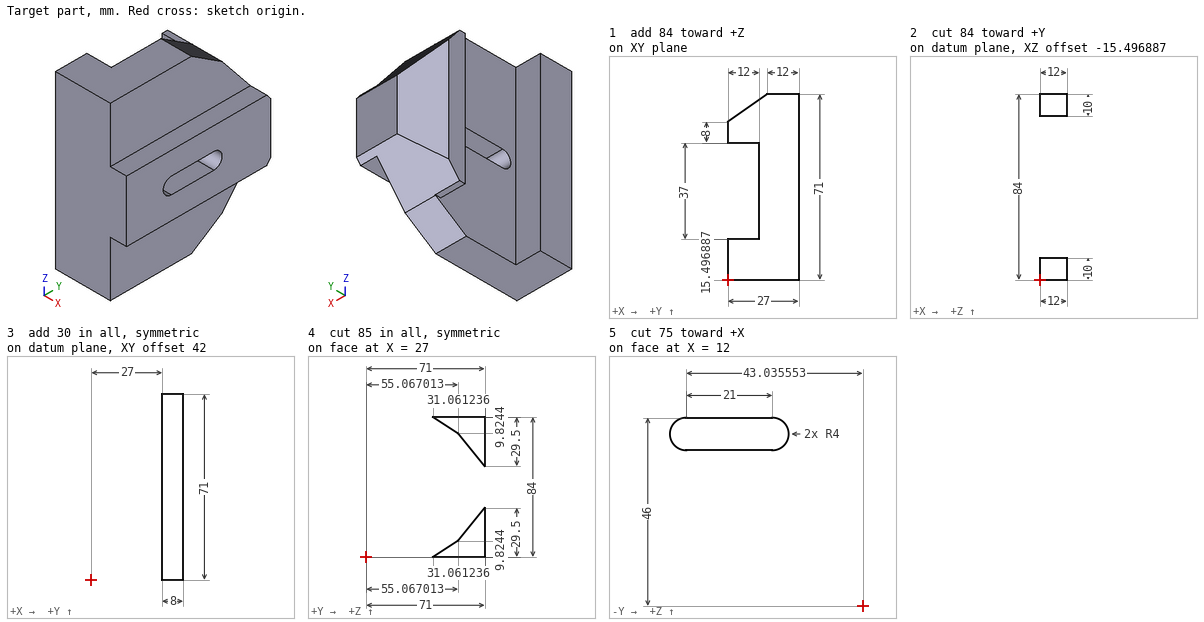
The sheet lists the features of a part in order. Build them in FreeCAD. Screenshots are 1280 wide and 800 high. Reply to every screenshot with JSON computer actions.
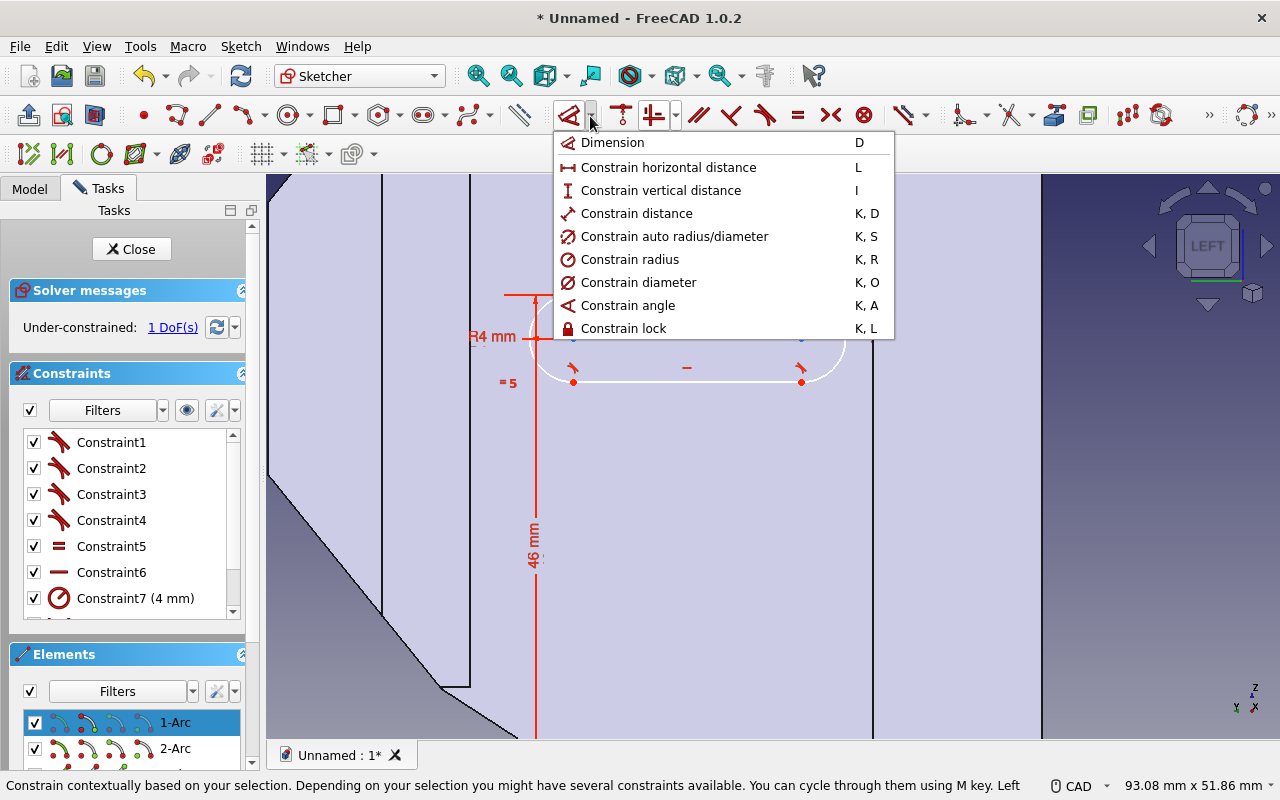
{"action": "left_click", "coordinate": [724, 168]}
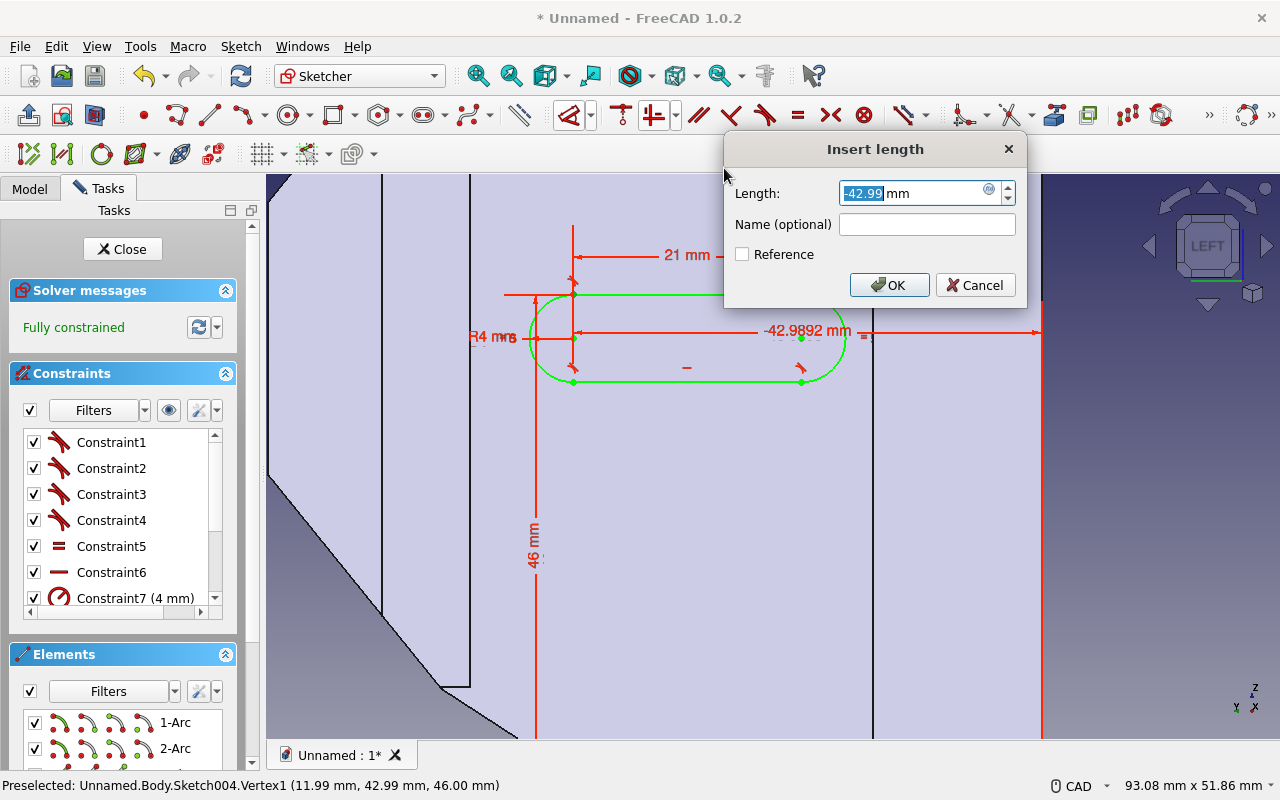
{"action": "type", "text": "-43.035553"}
{"action": "key", "text": "Return"}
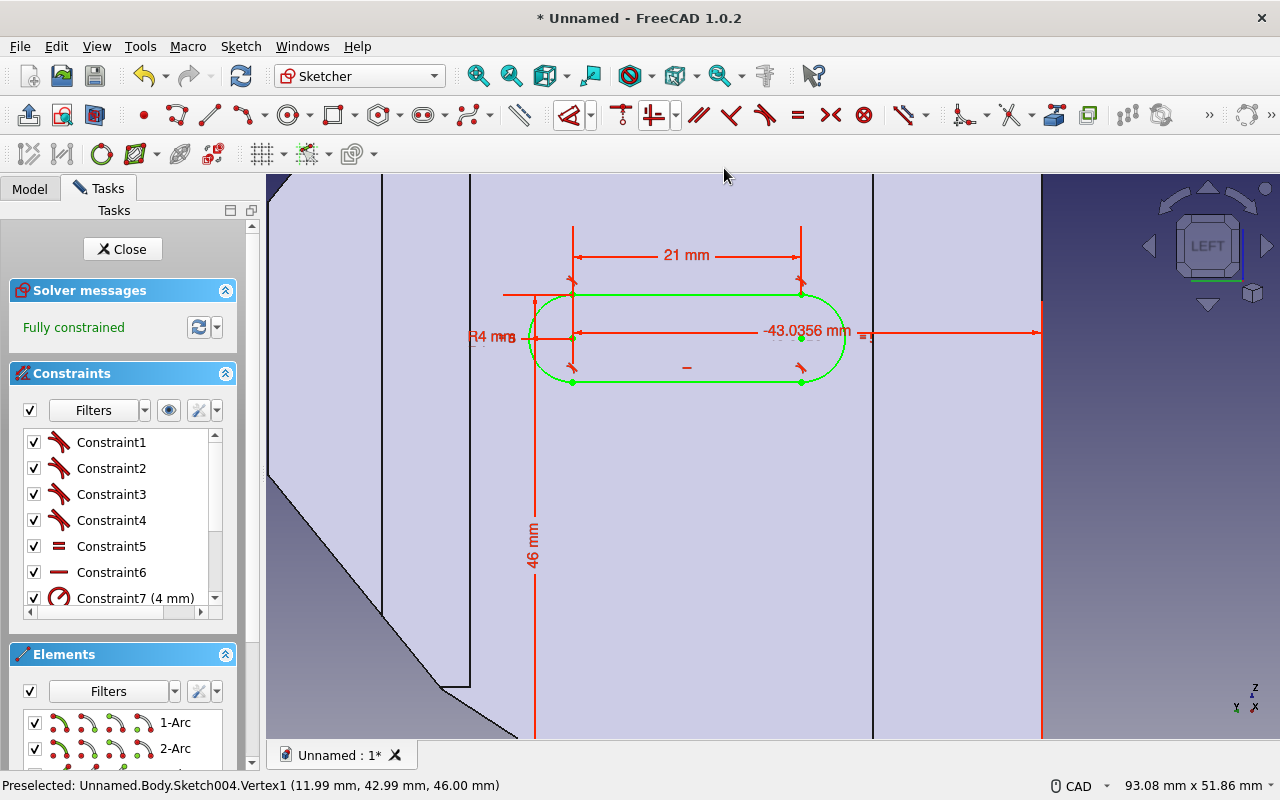
{"action": "left_click", "coordinate": [123, 249]}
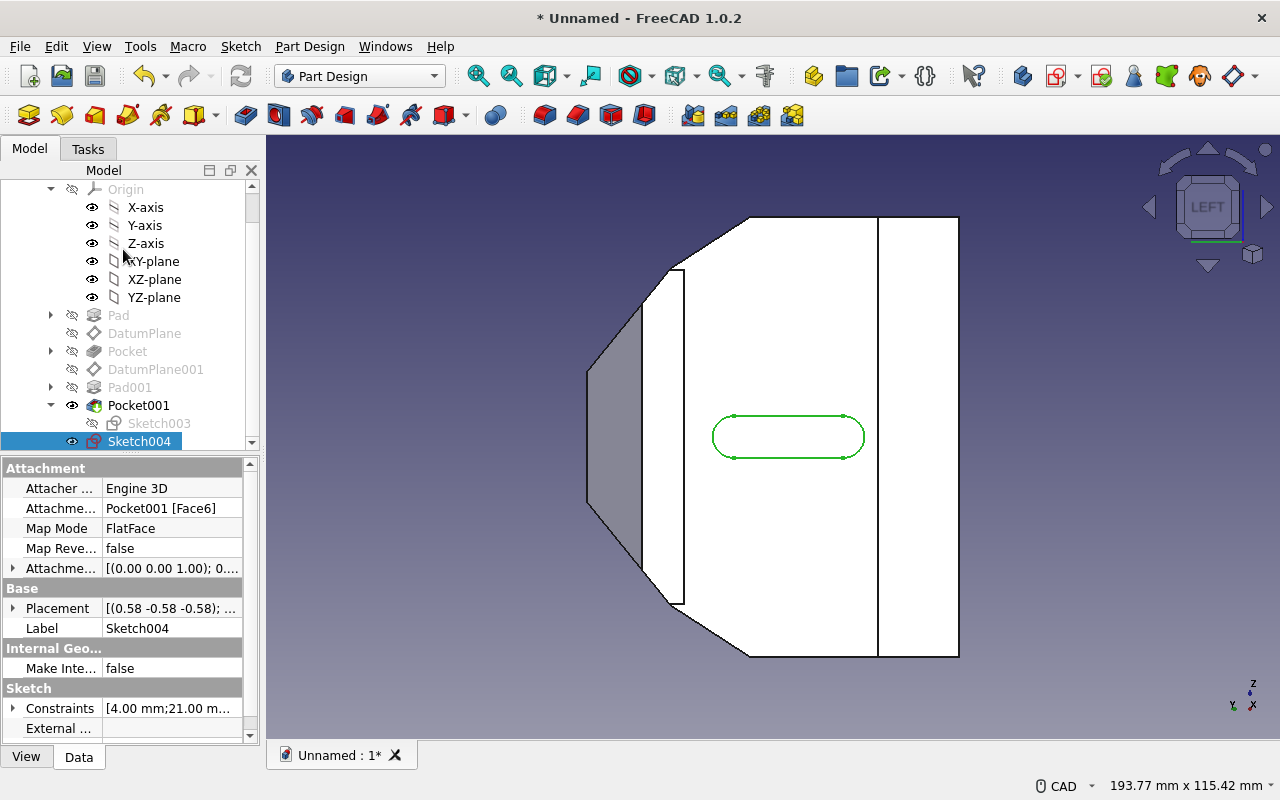
{"action": "left_click", "coordinate": [246, 116]}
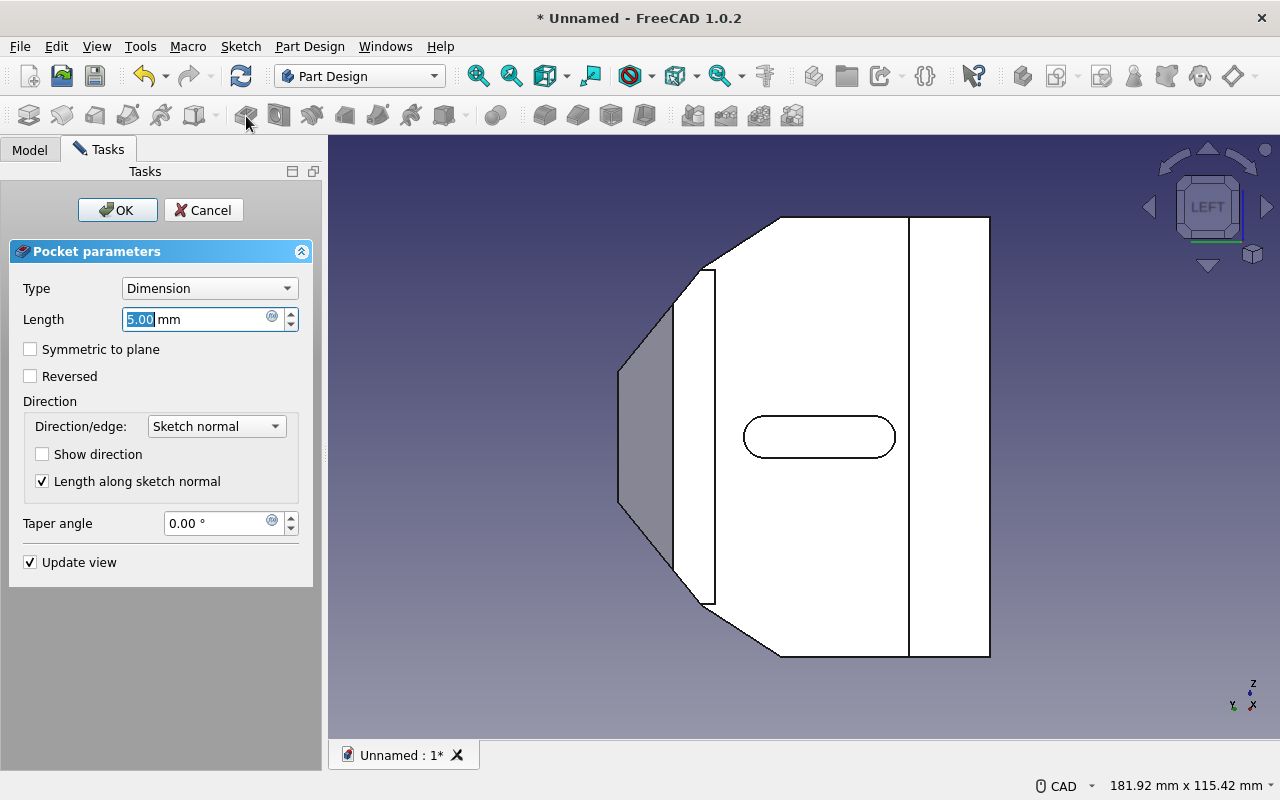
{"action": "type", "text": "75"}
{"action": "key", "text": "Tab"}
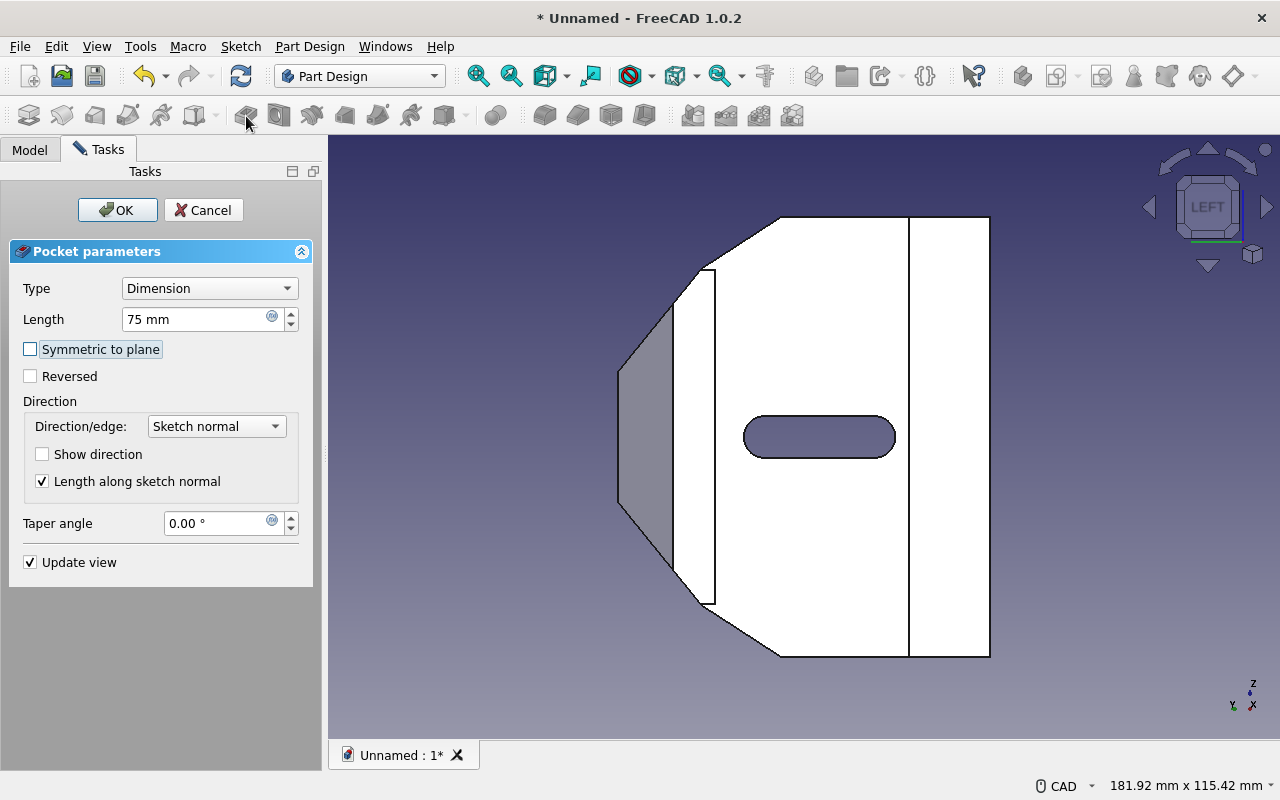
{"action": "left_click", "coordinate": [118, 210]}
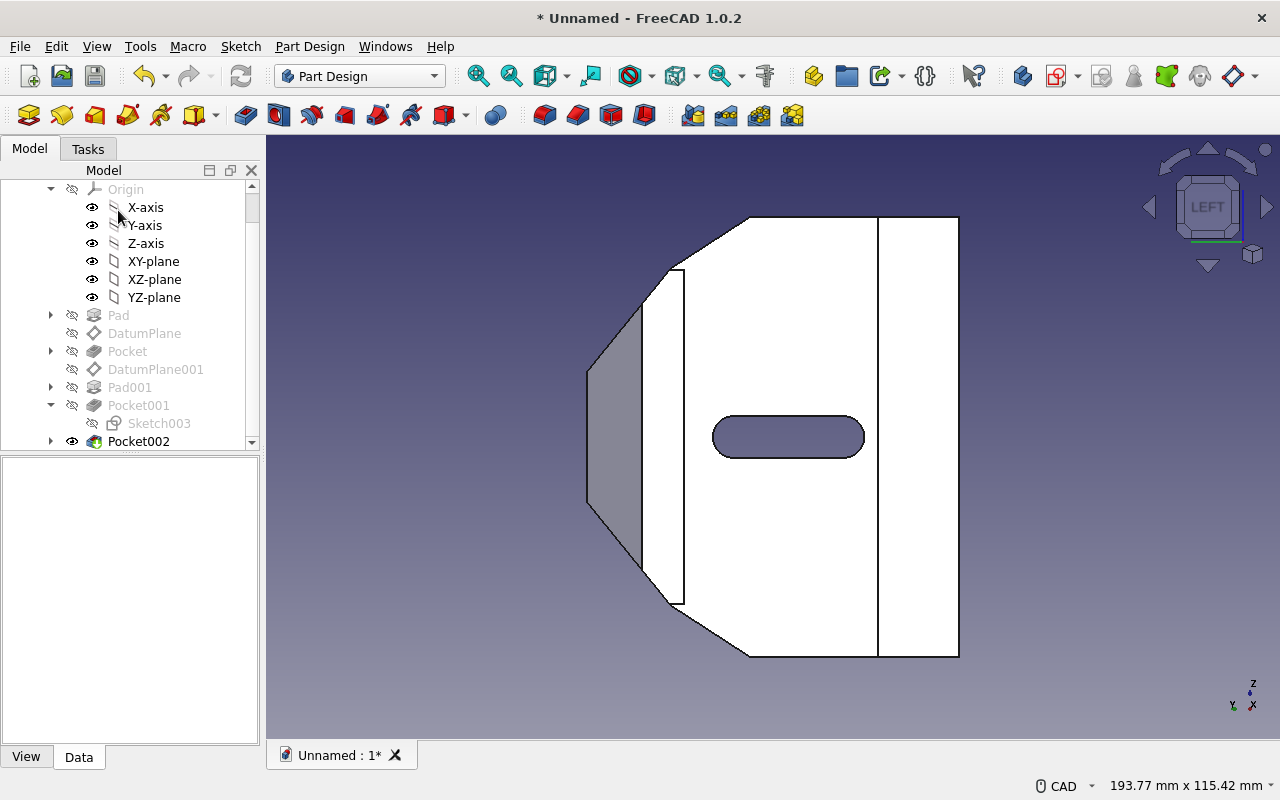
{"action": "key", "text": "0"}